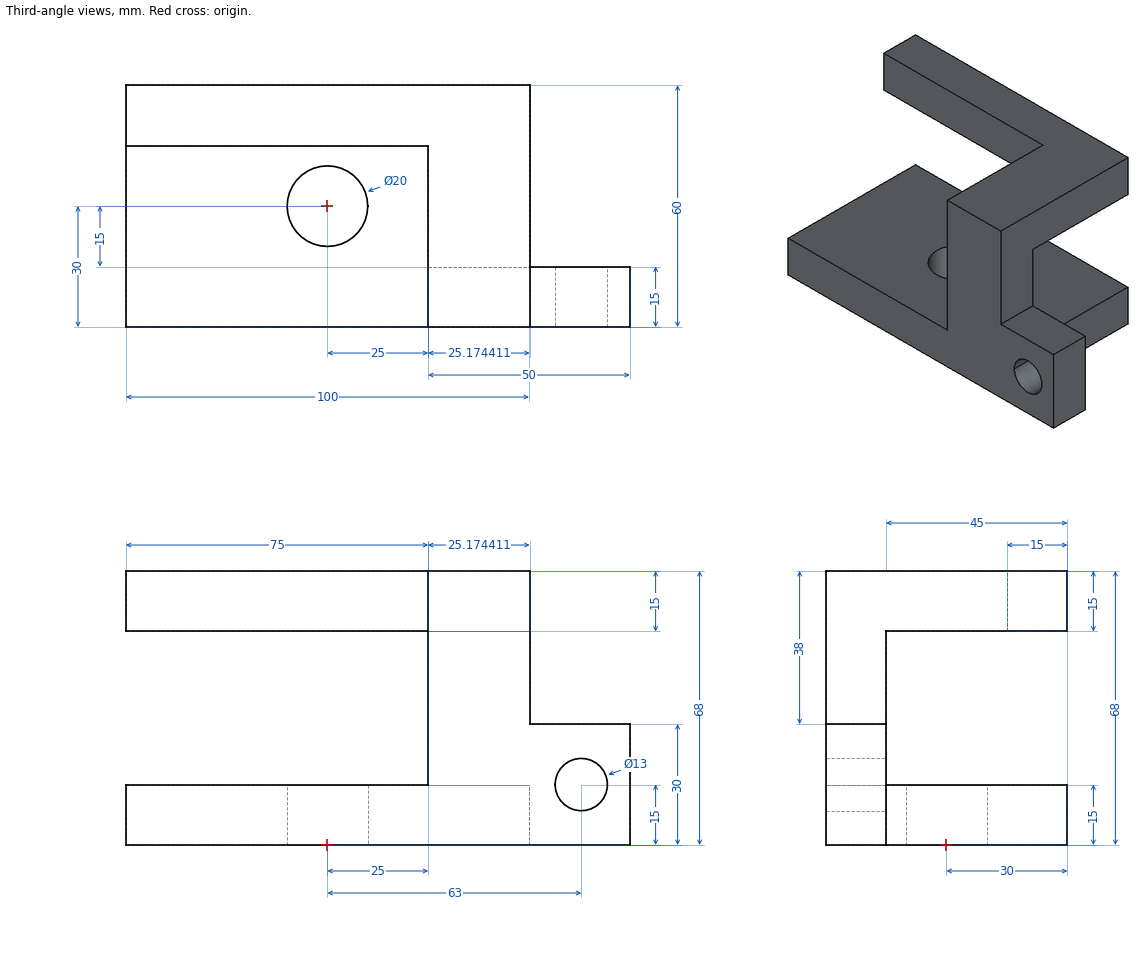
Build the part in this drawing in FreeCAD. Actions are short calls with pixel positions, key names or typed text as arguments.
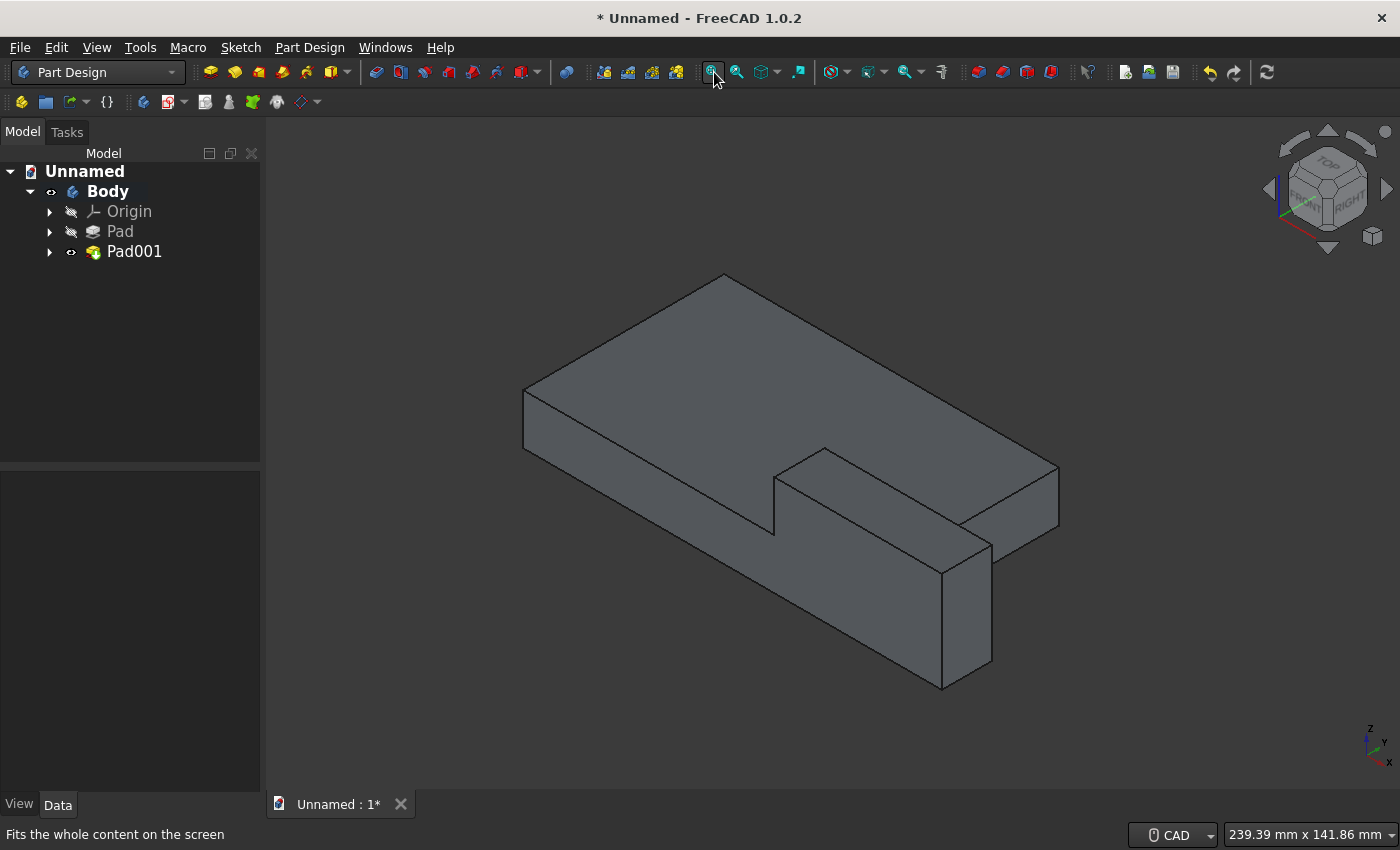
click(931, 538)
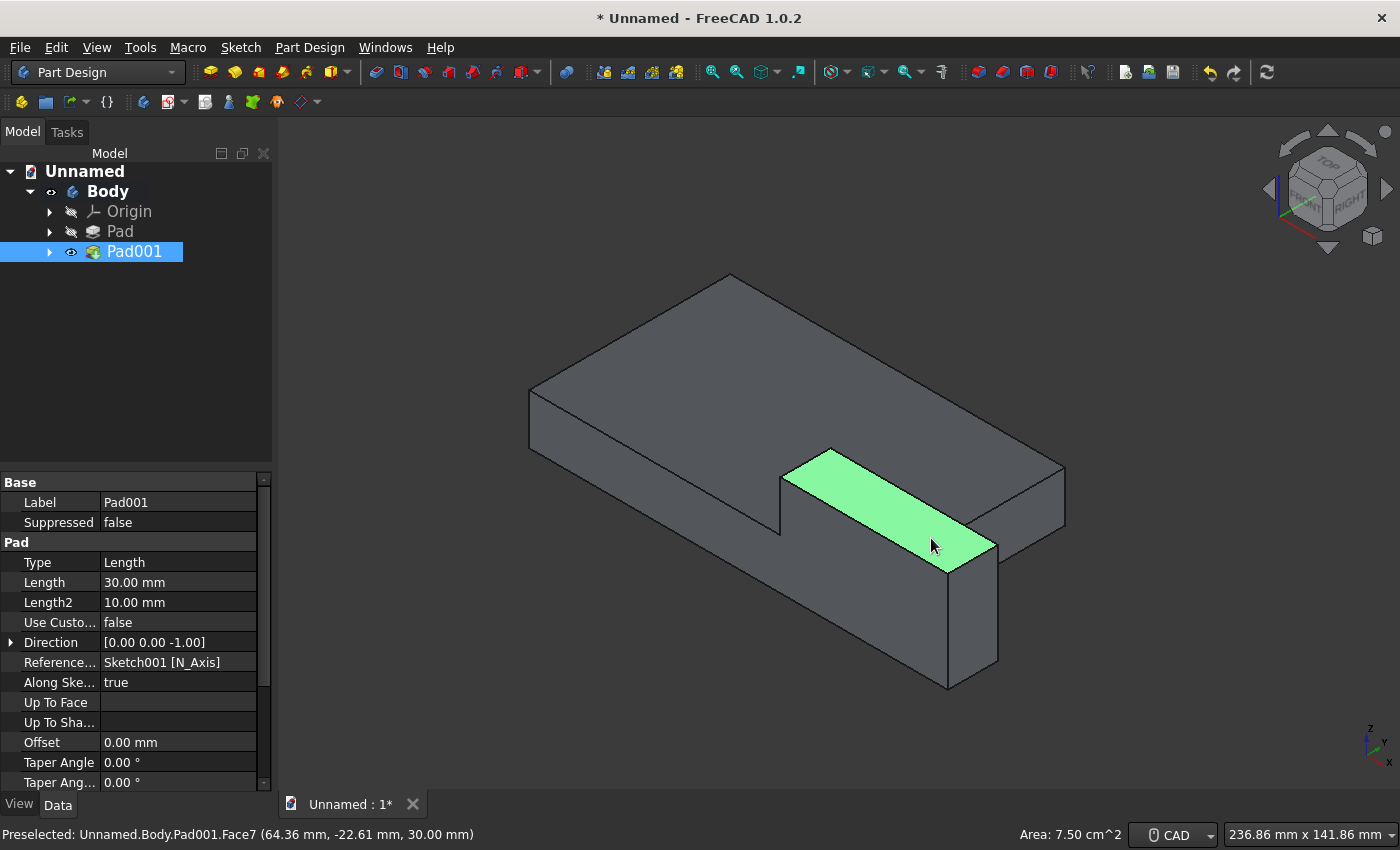
click(168, 102)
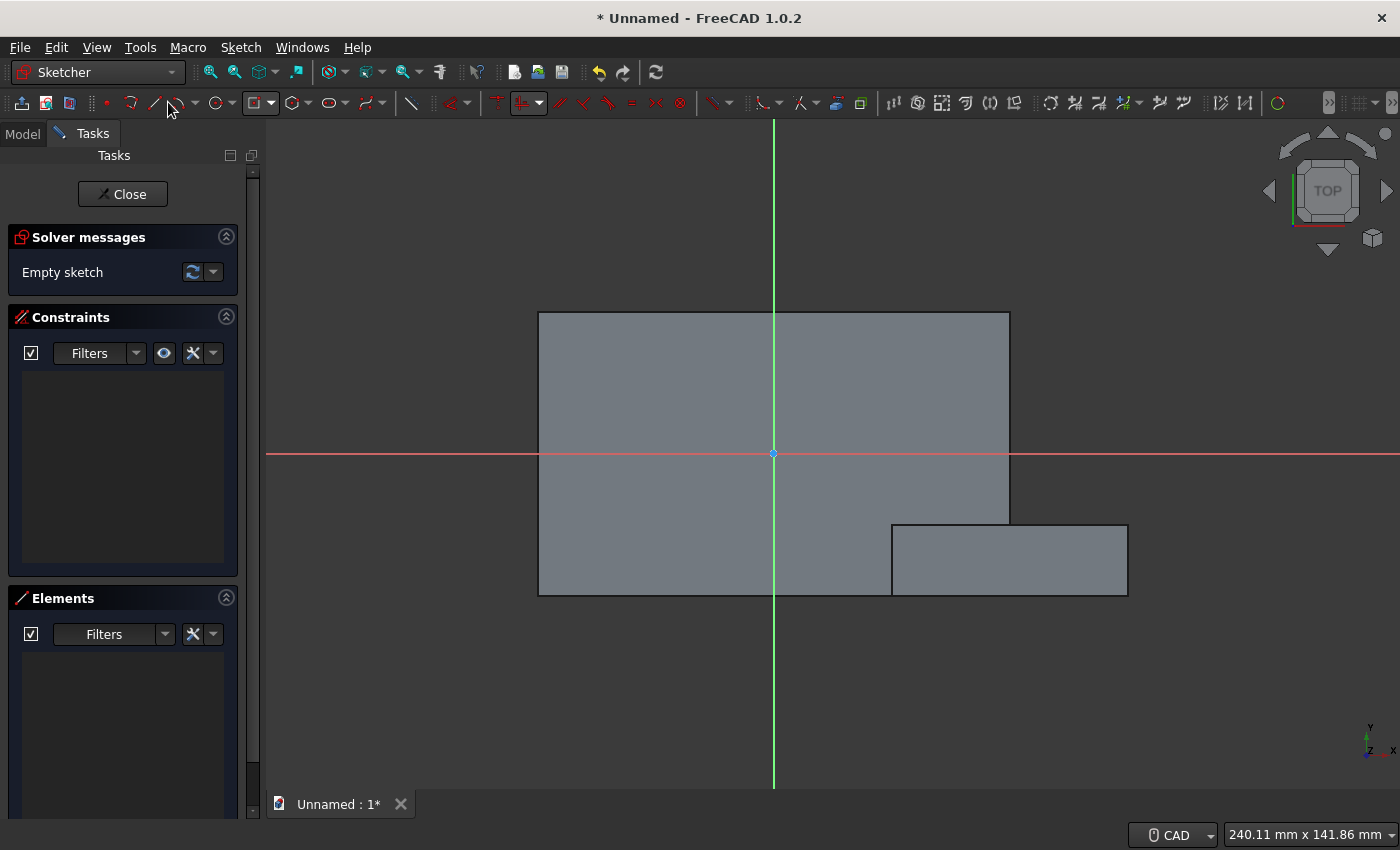
scroll(967, 566, up, 5)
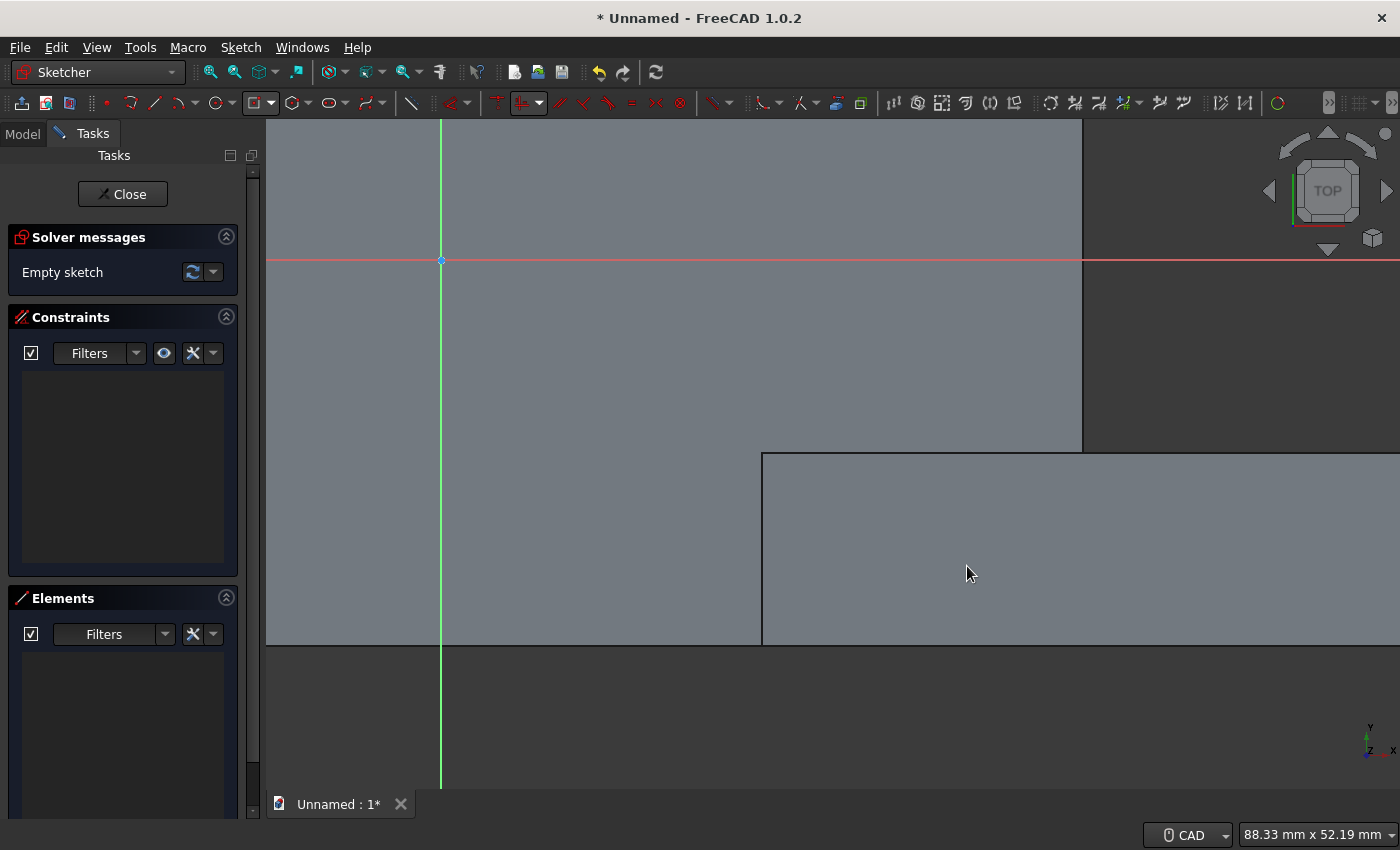
click(274, 104)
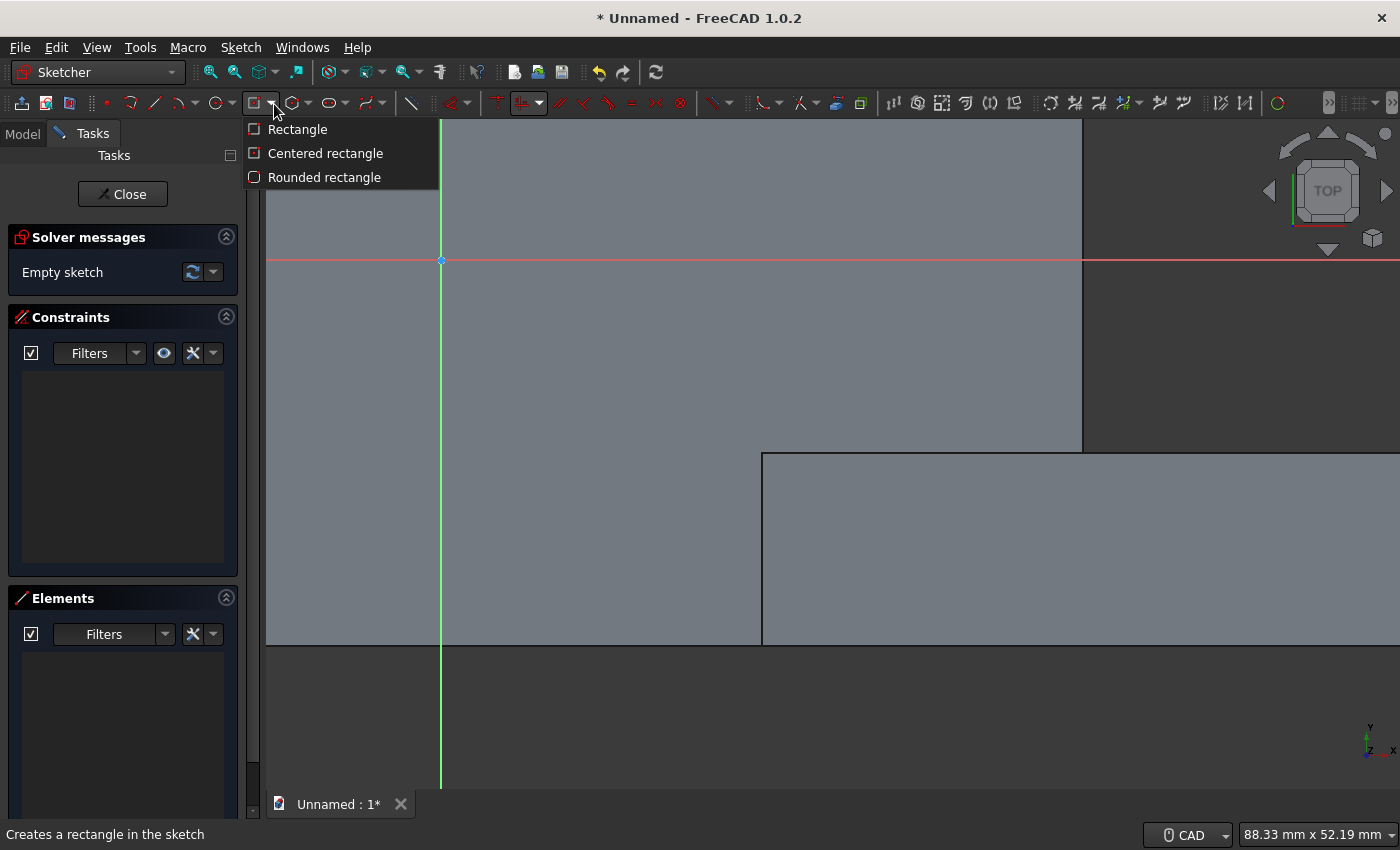
click(340, 129)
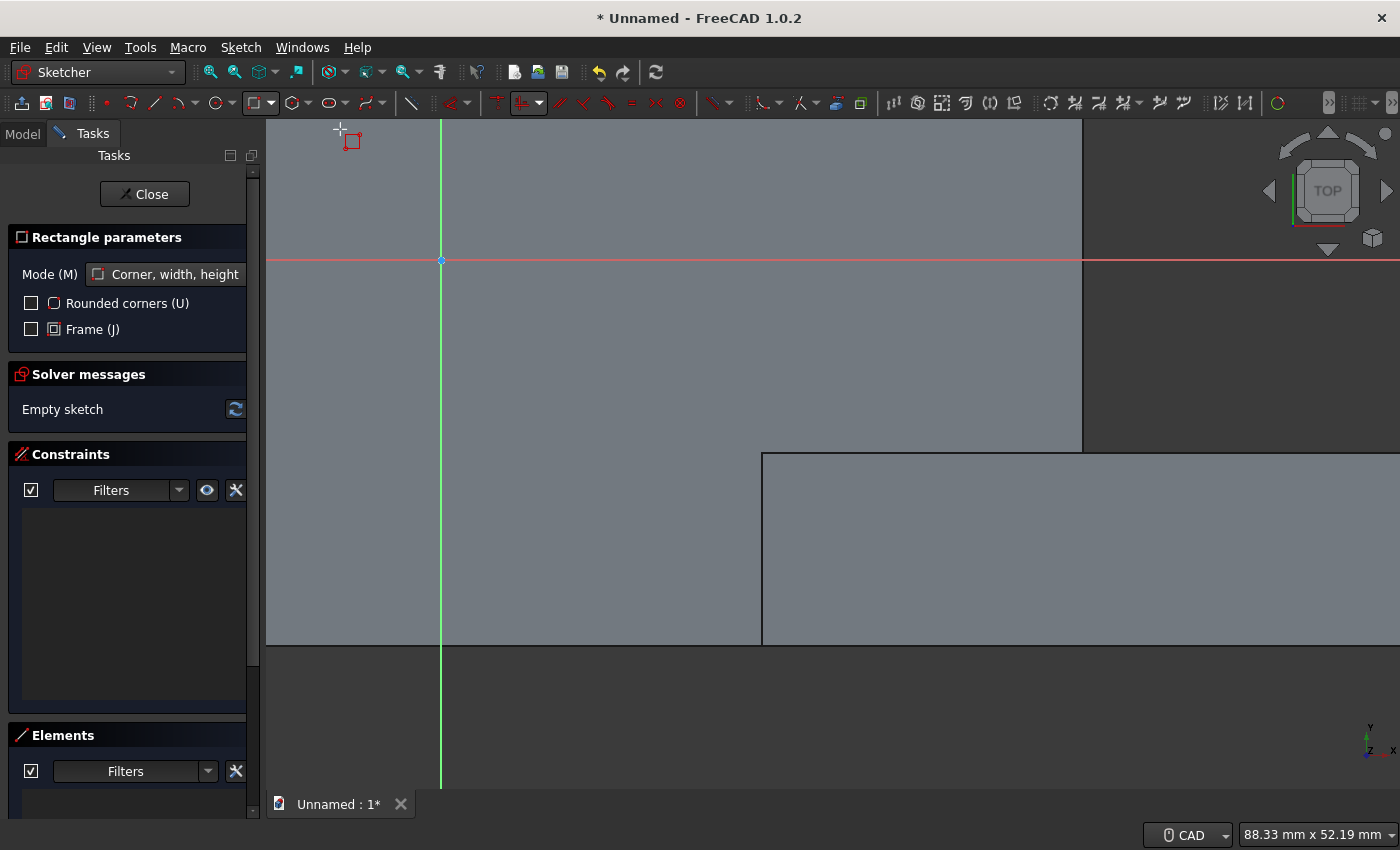
click(762, 453)
move(1085, 646)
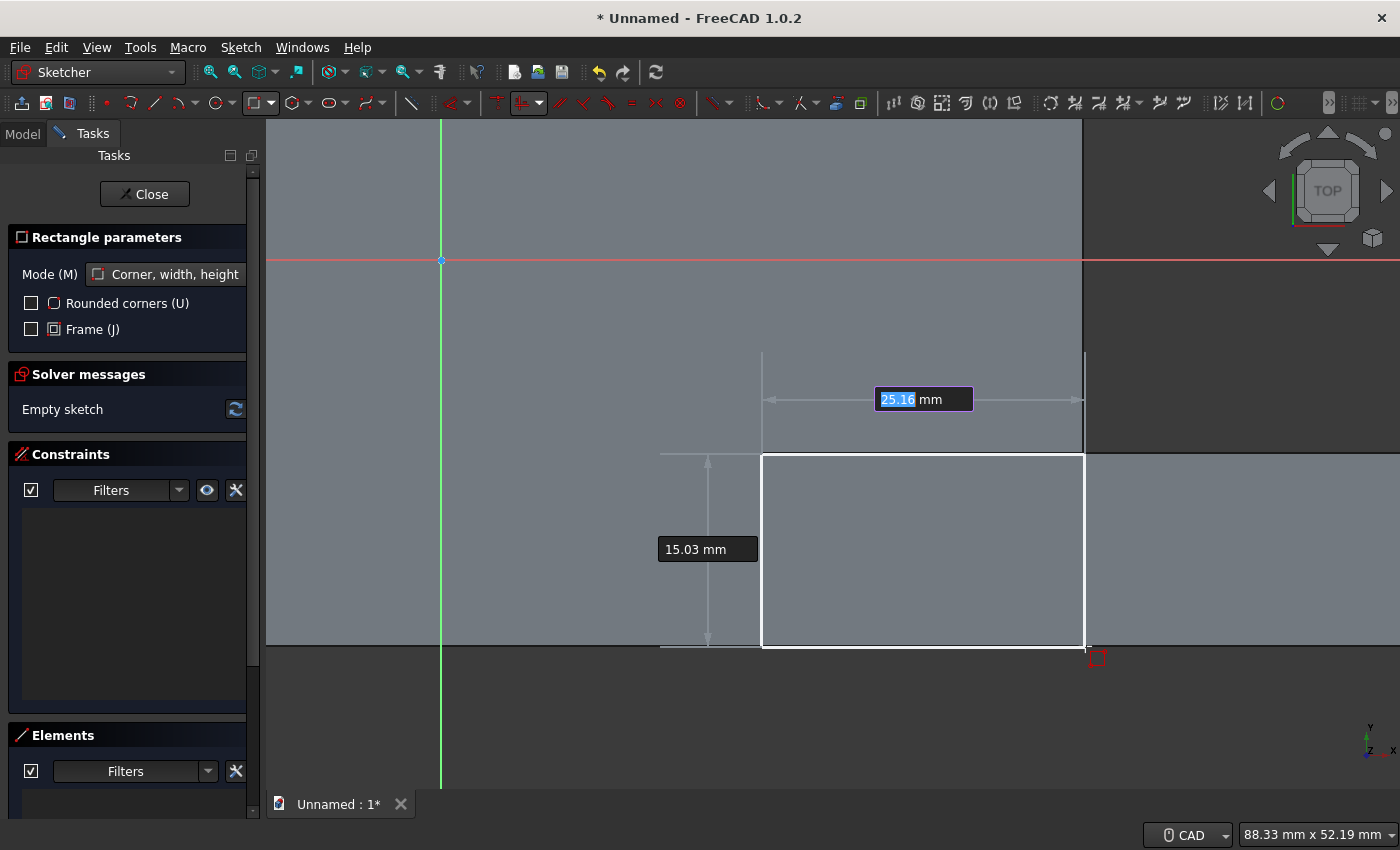
text(25.174411)
key(Tab)
text(15)
key(Return)
key(Escape)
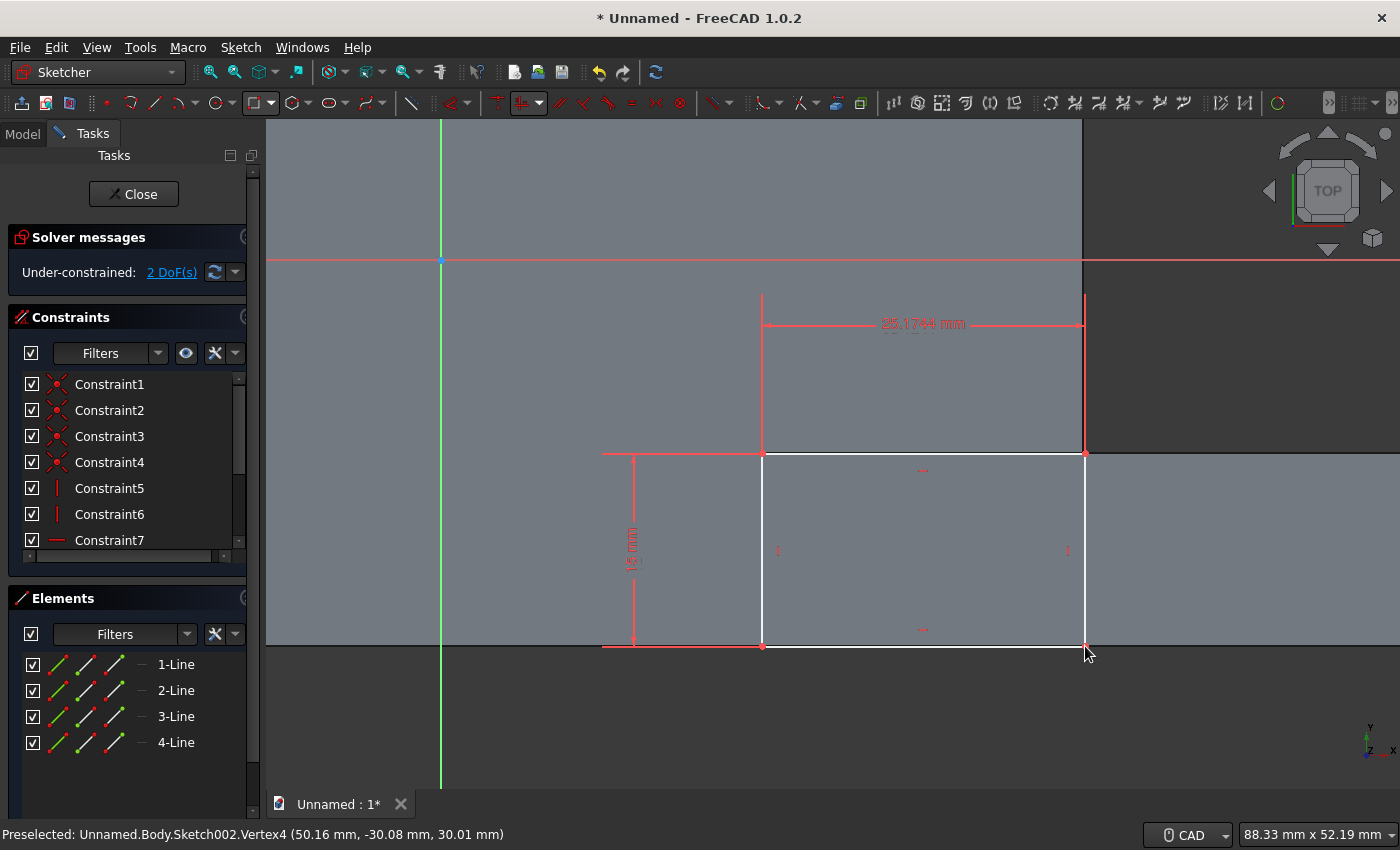
click(450, 104)